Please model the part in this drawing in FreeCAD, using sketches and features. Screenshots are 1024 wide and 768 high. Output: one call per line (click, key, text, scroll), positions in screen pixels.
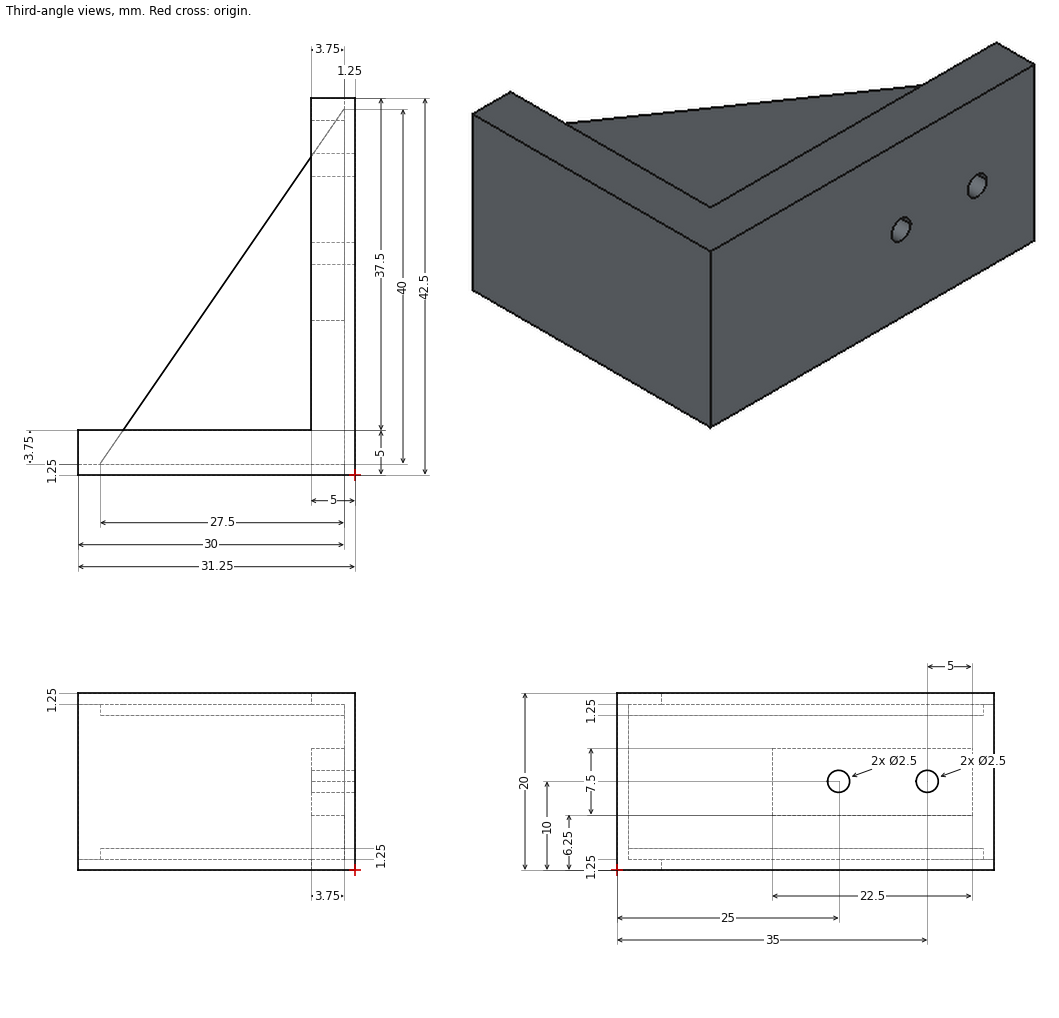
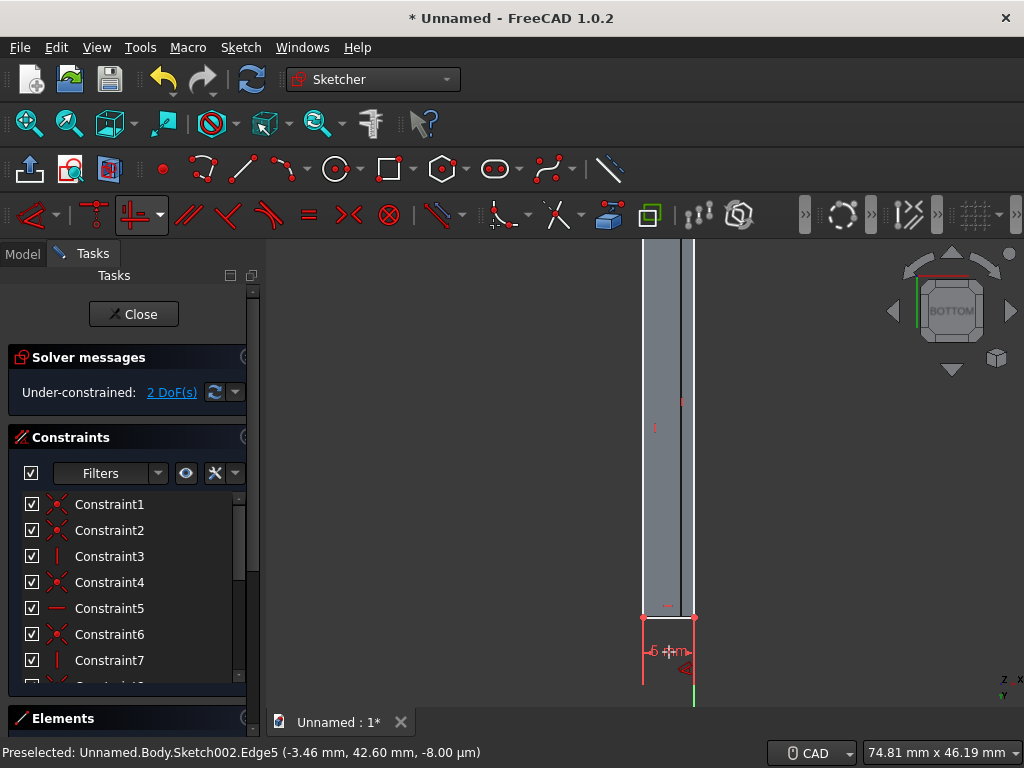
click(643, 351)
click(677, 442)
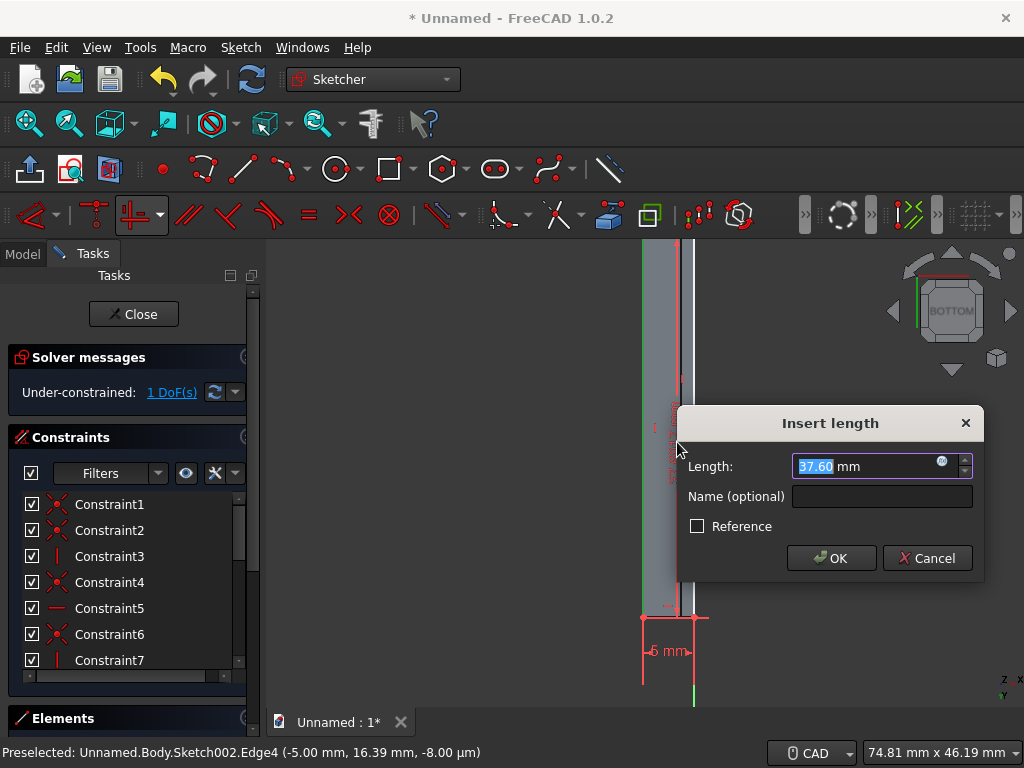
text(37.5)
key(Return)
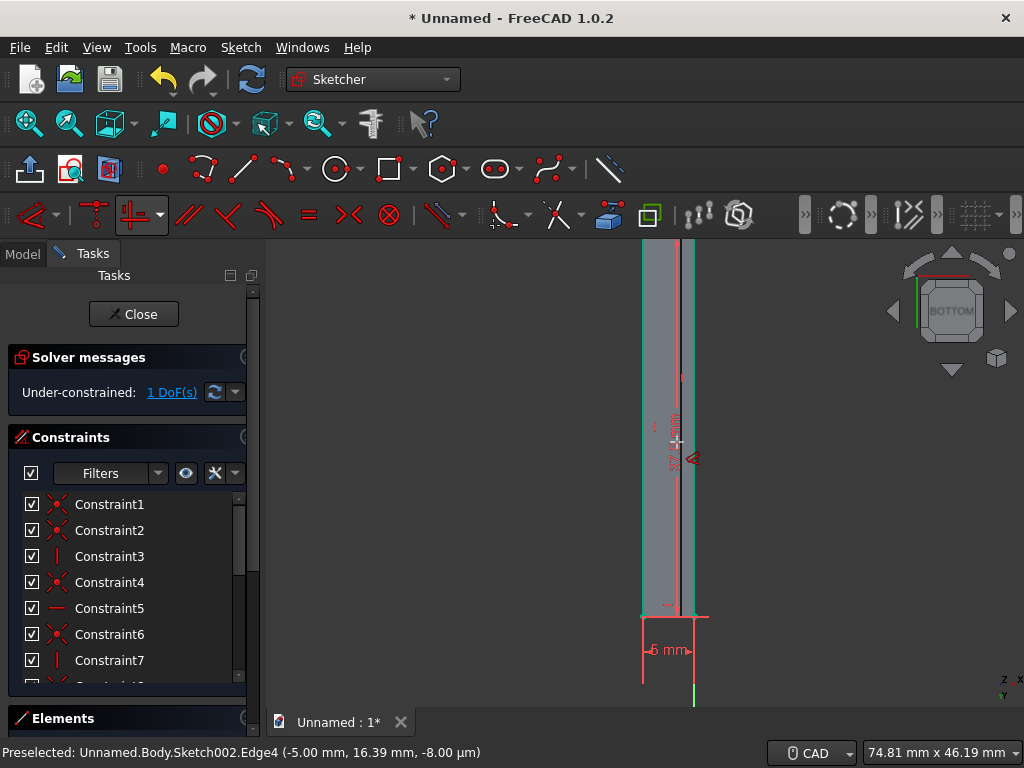
scroll(659, 619, down, 2)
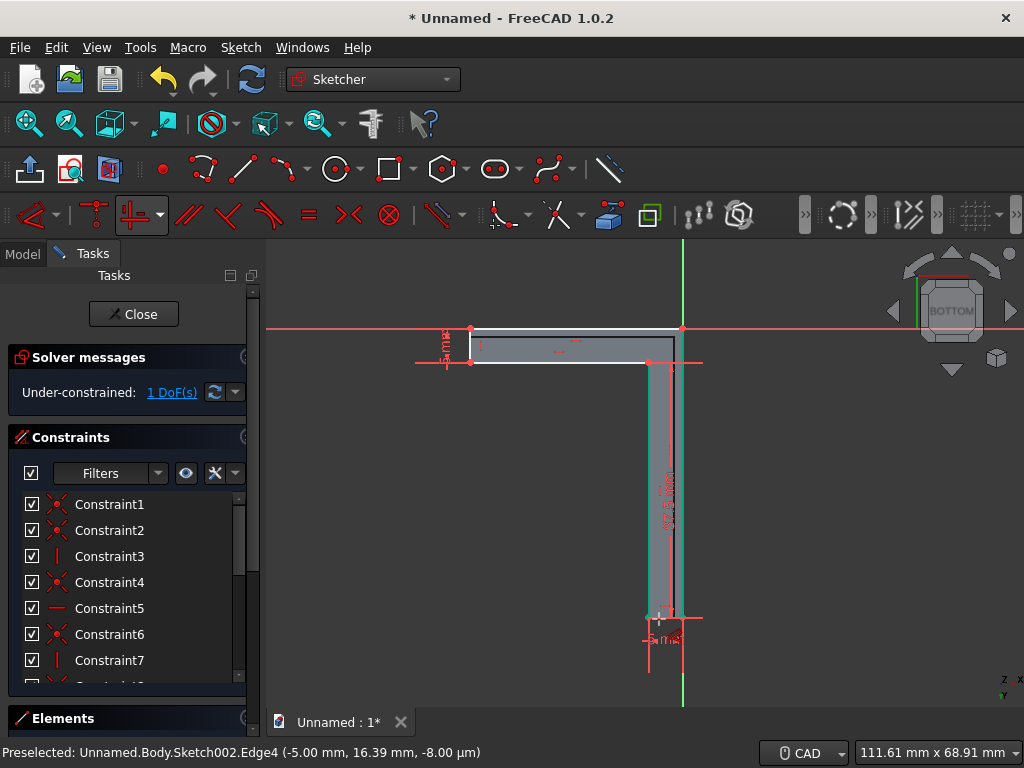
click(619, 329)
click(576, 295)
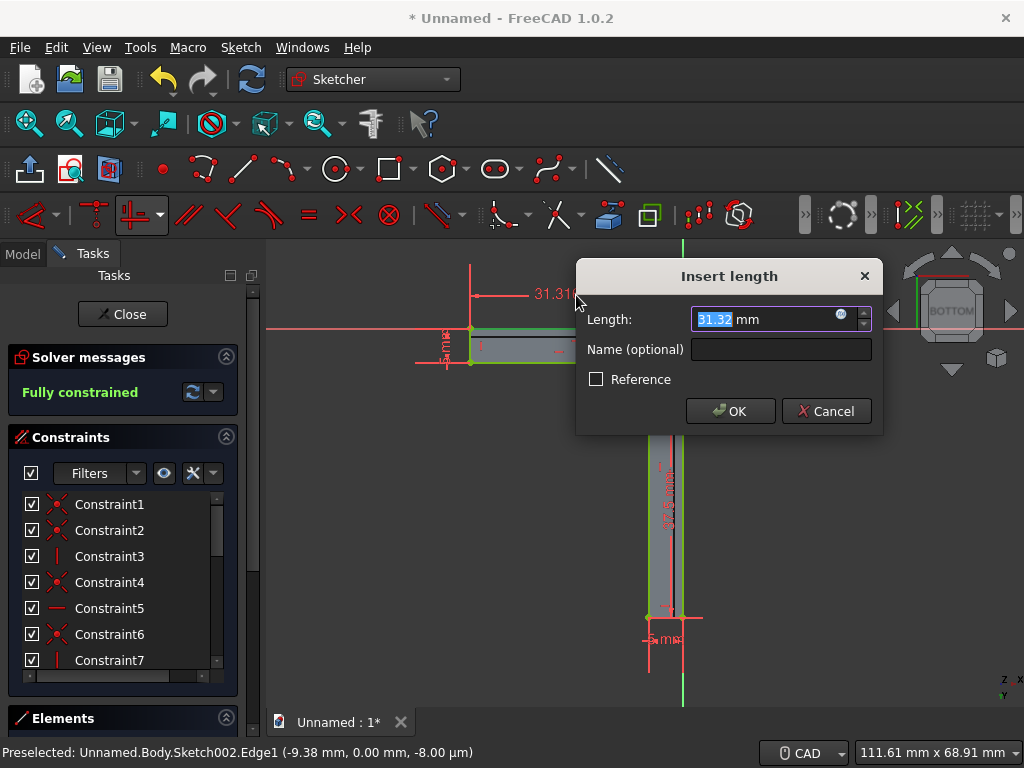
text(31.25)
key(Return)
key(Escape)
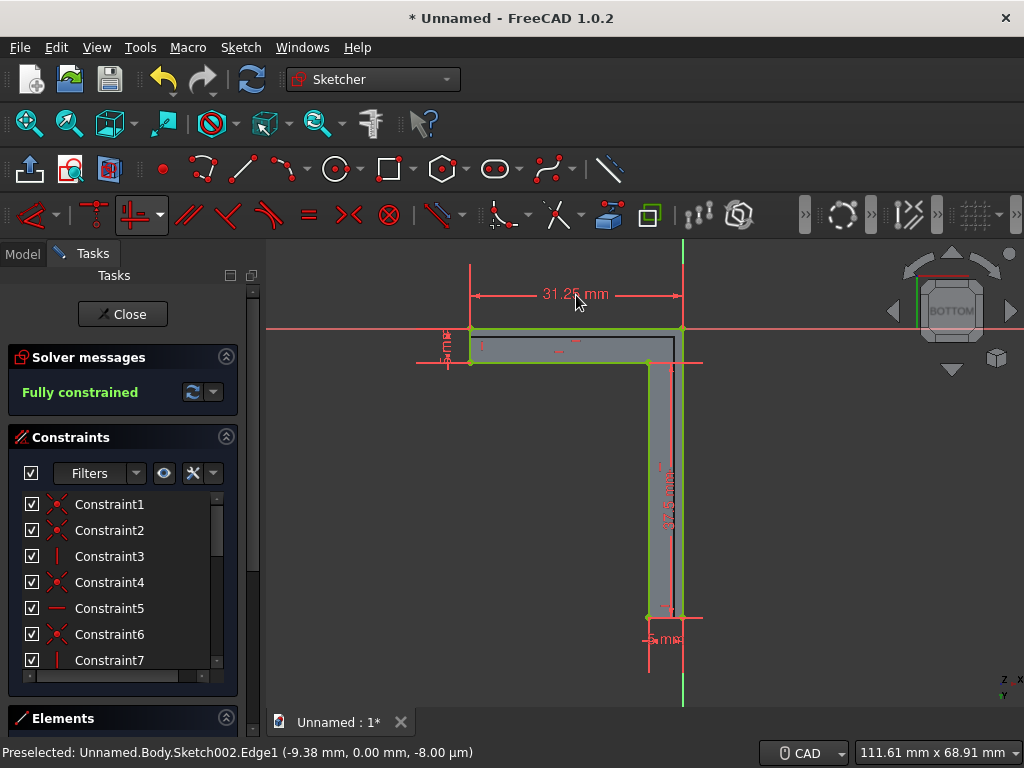
click(123, 314)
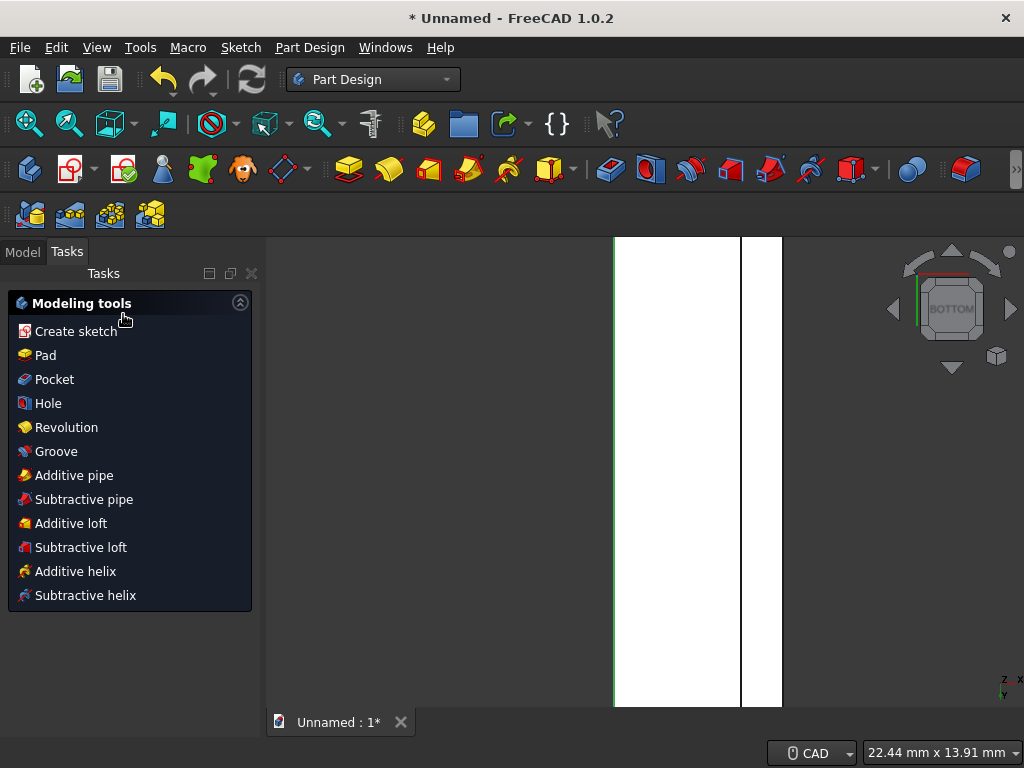
click(350, 170)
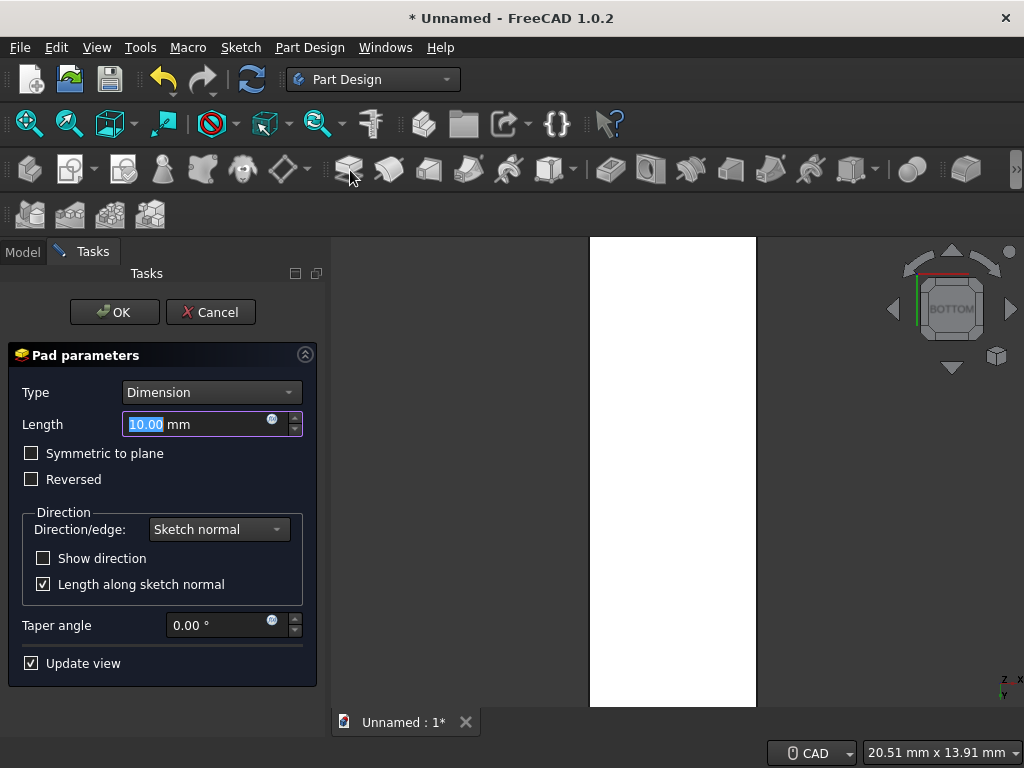
text(1.25)
key(Tab)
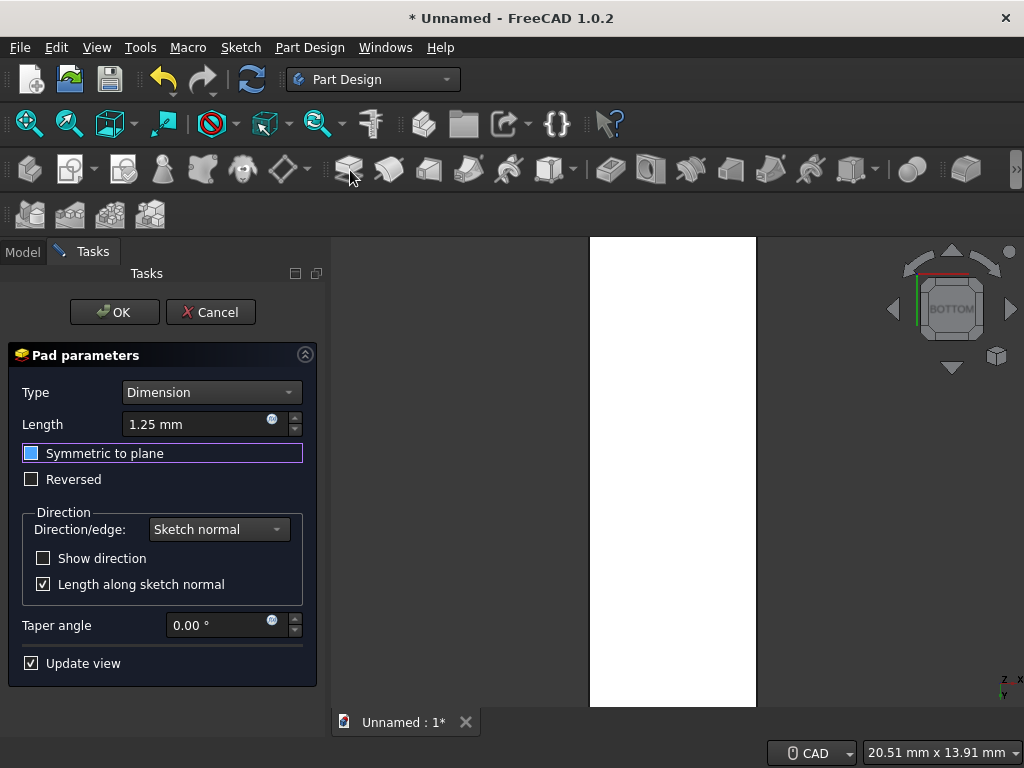
click(30, 479)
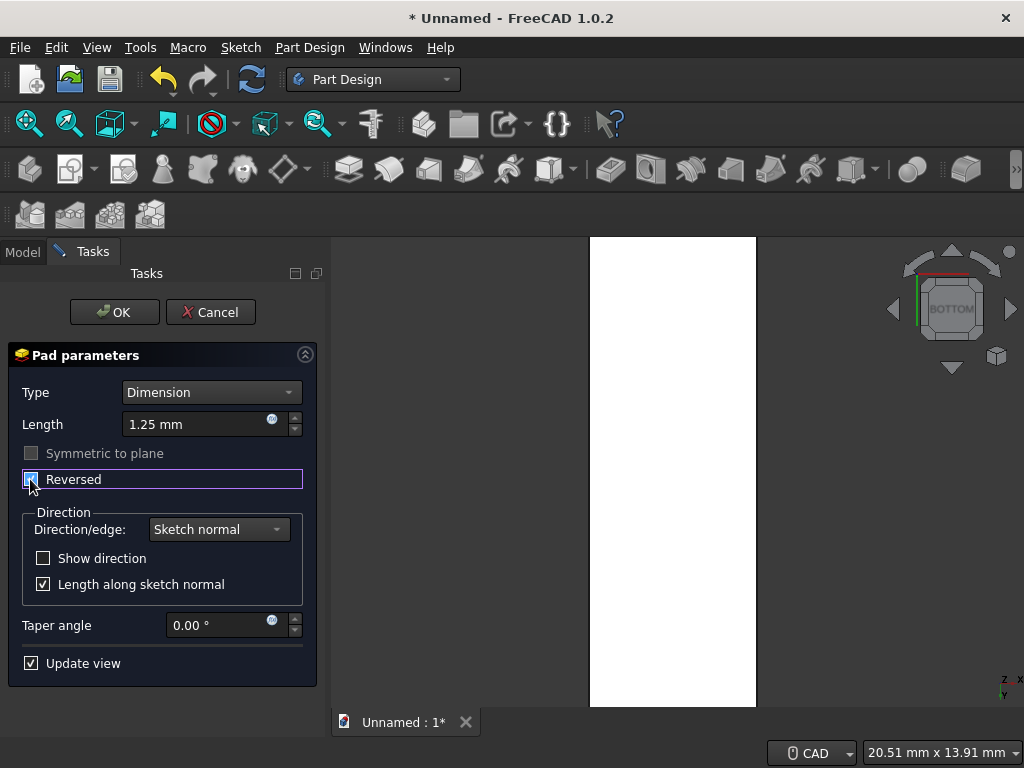
click(115, 312)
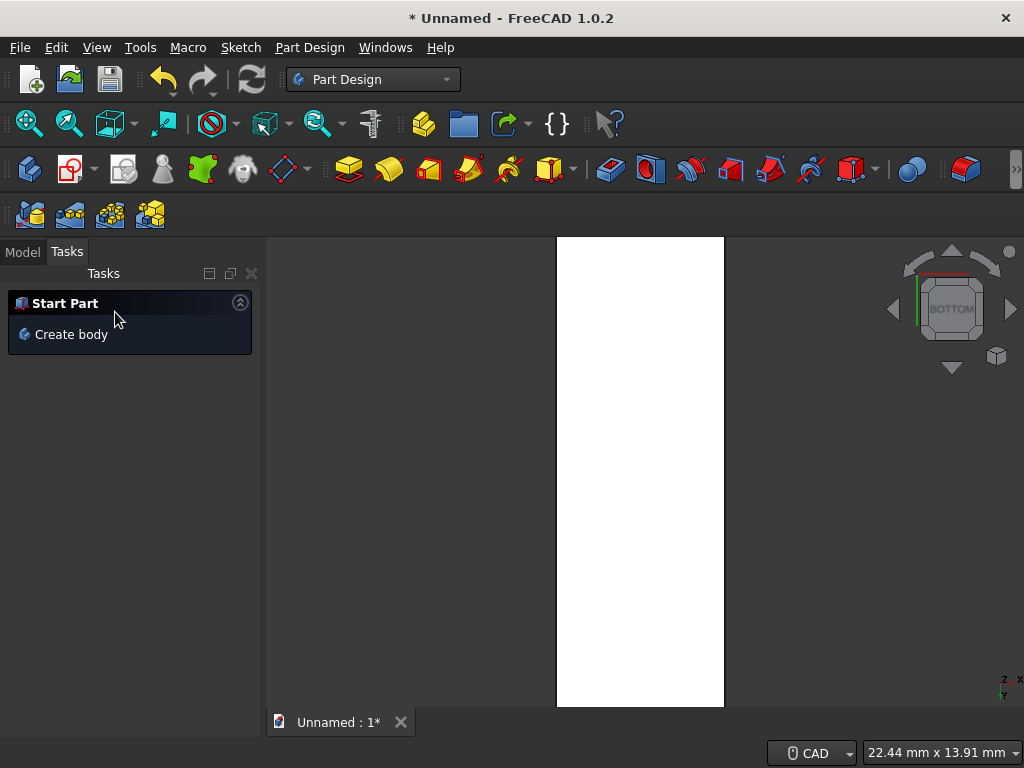
click(30, 124)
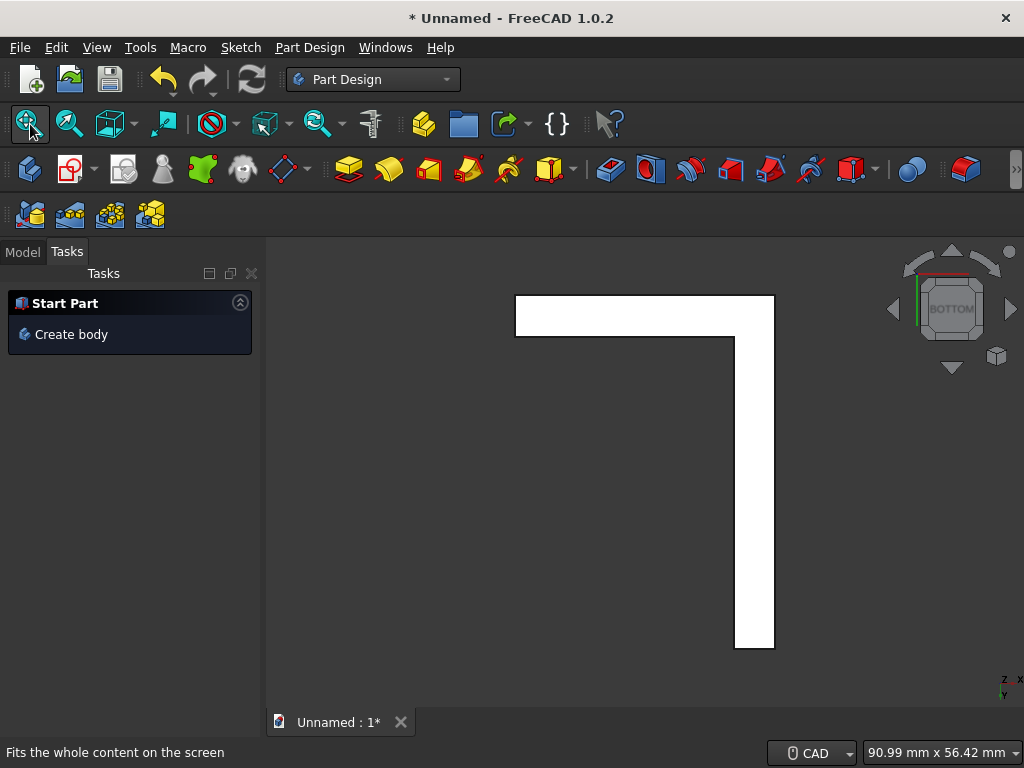
click(23, 251)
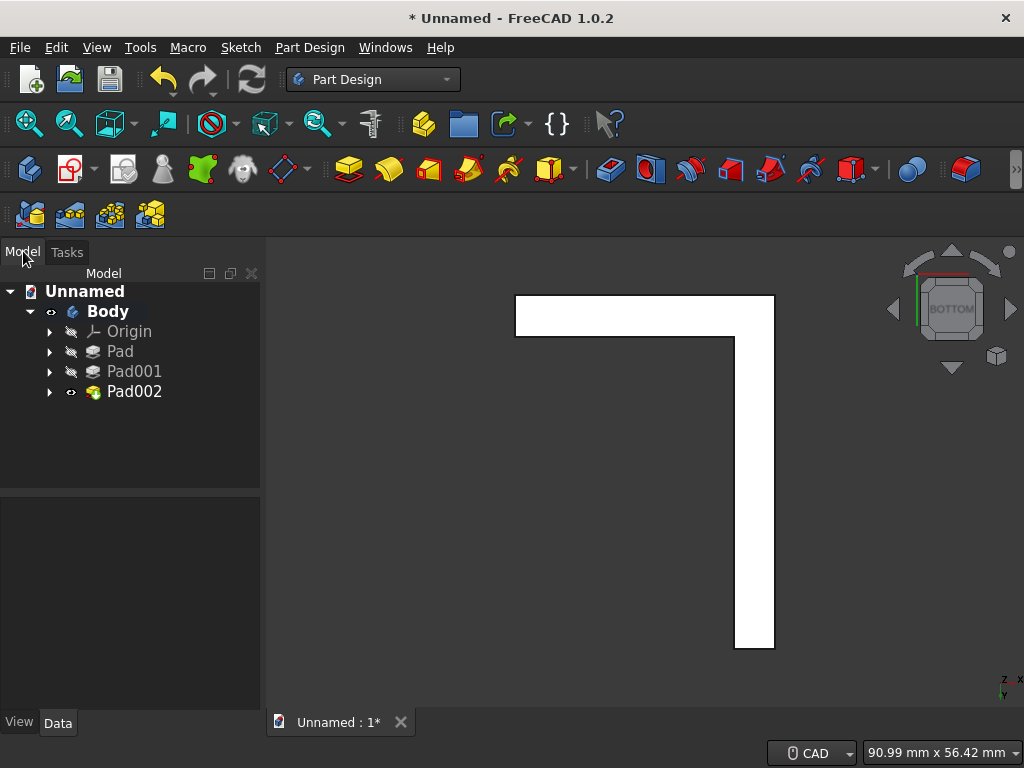
click(50, 332)